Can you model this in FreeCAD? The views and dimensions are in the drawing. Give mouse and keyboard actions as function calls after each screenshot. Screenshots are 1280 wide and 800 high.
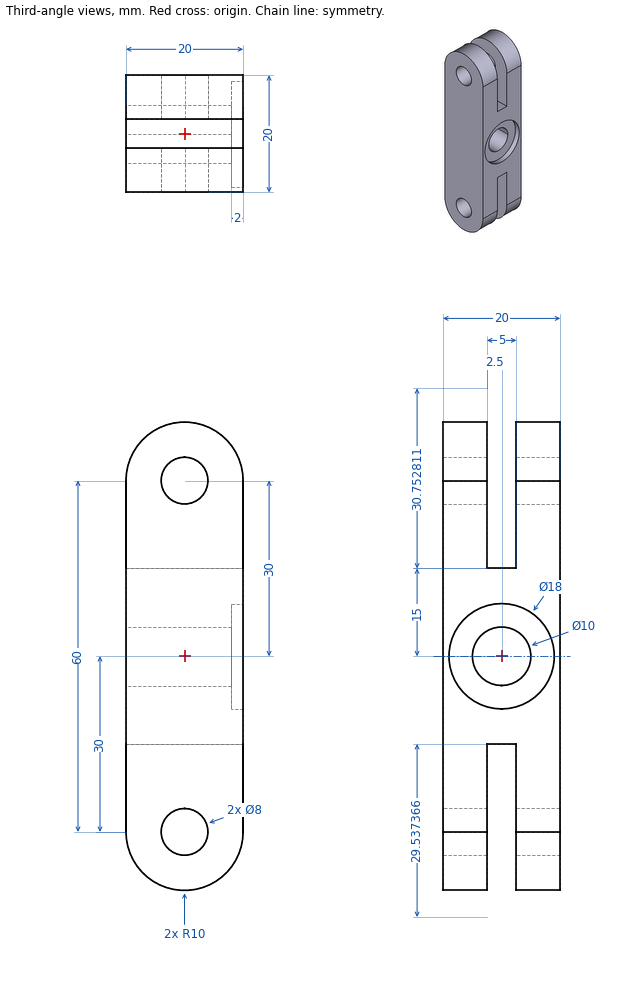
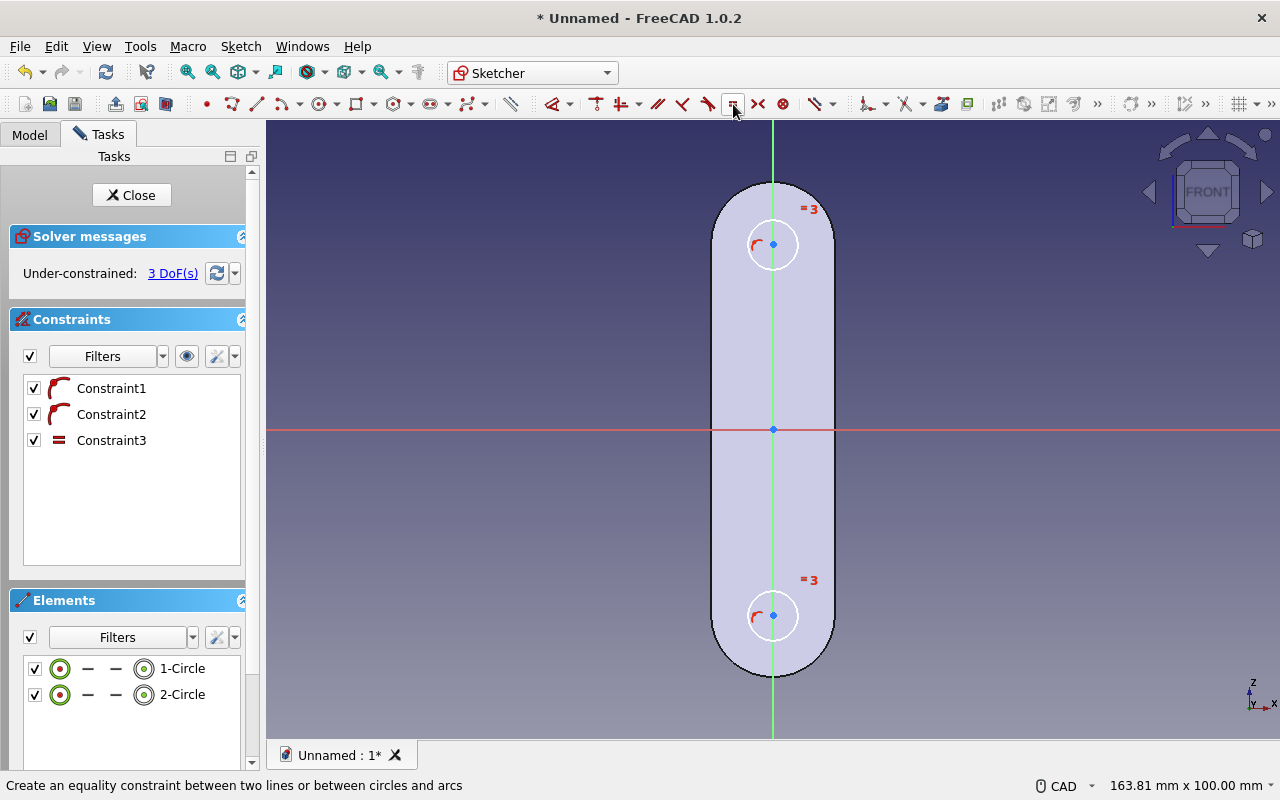
key(d)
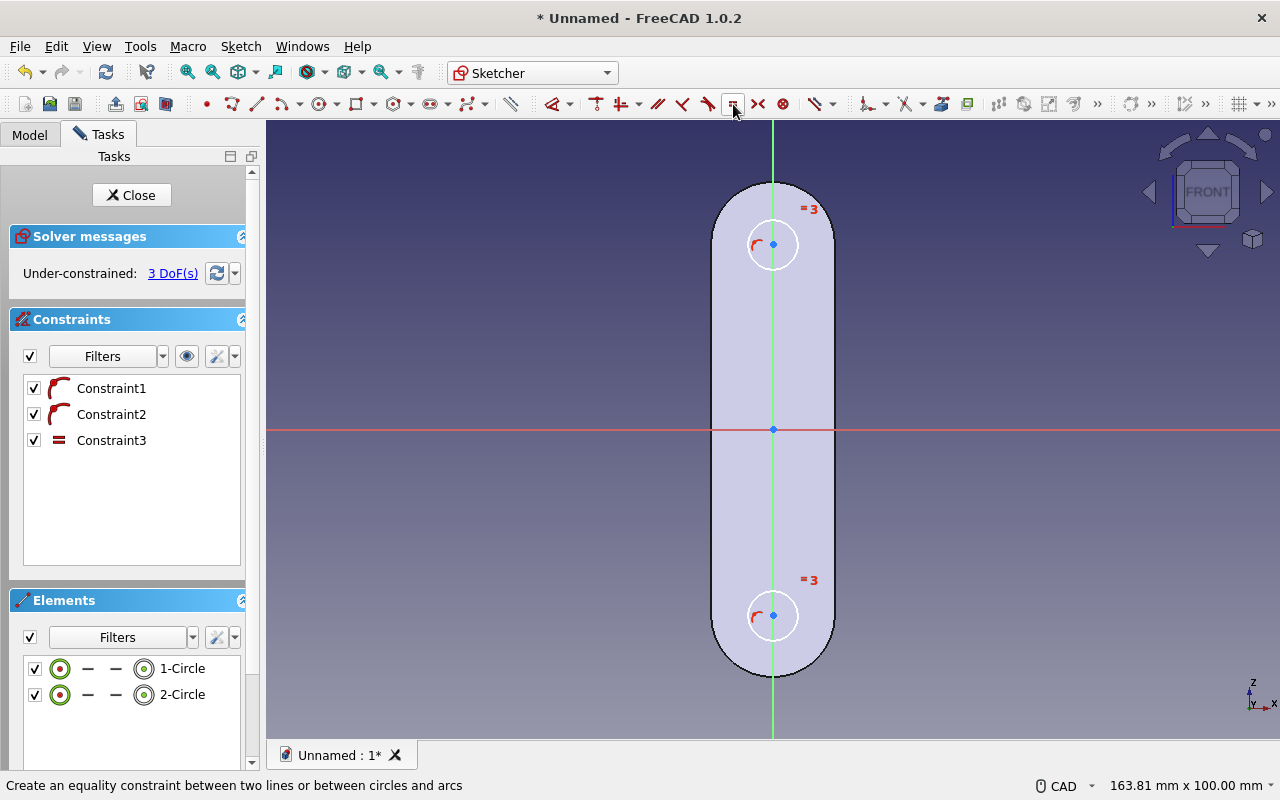
click(790, 598)
click(812, 575)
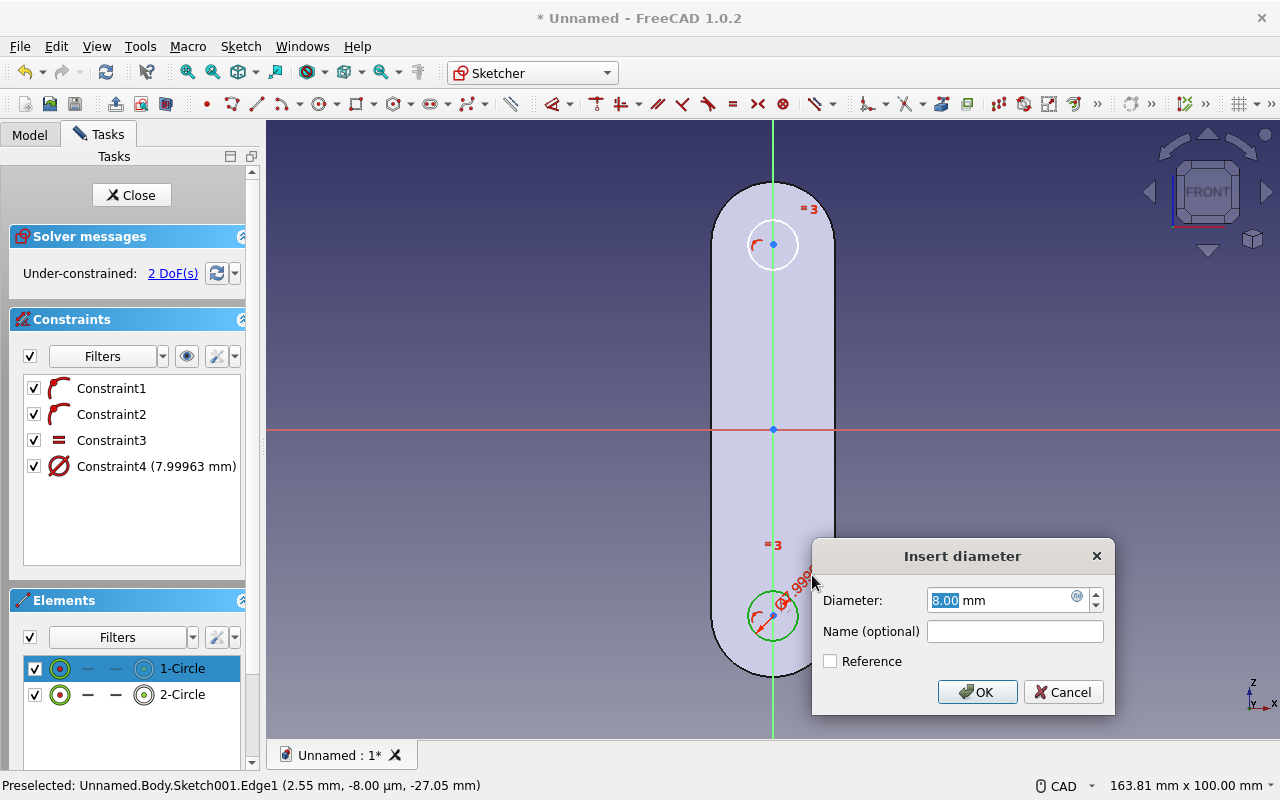
text(8)
key(Return)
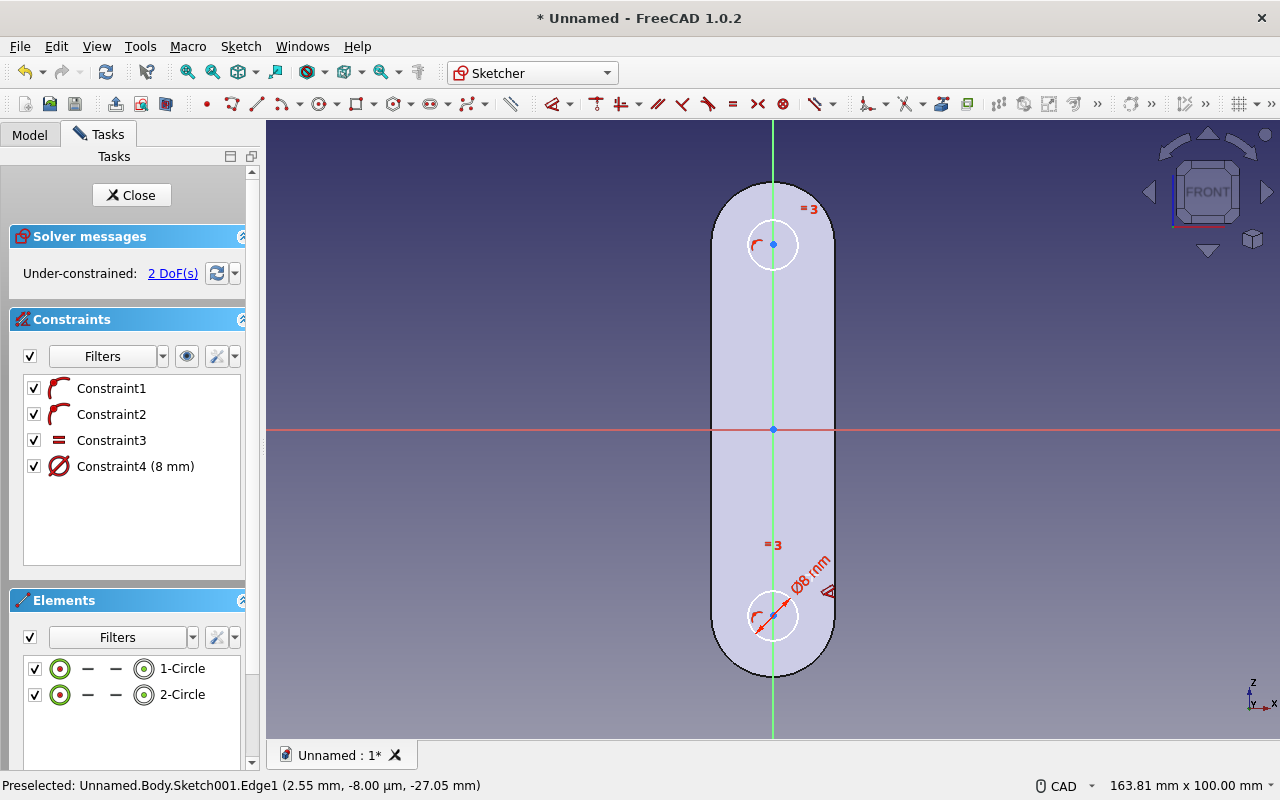
click(773, 616)
click(807, 523)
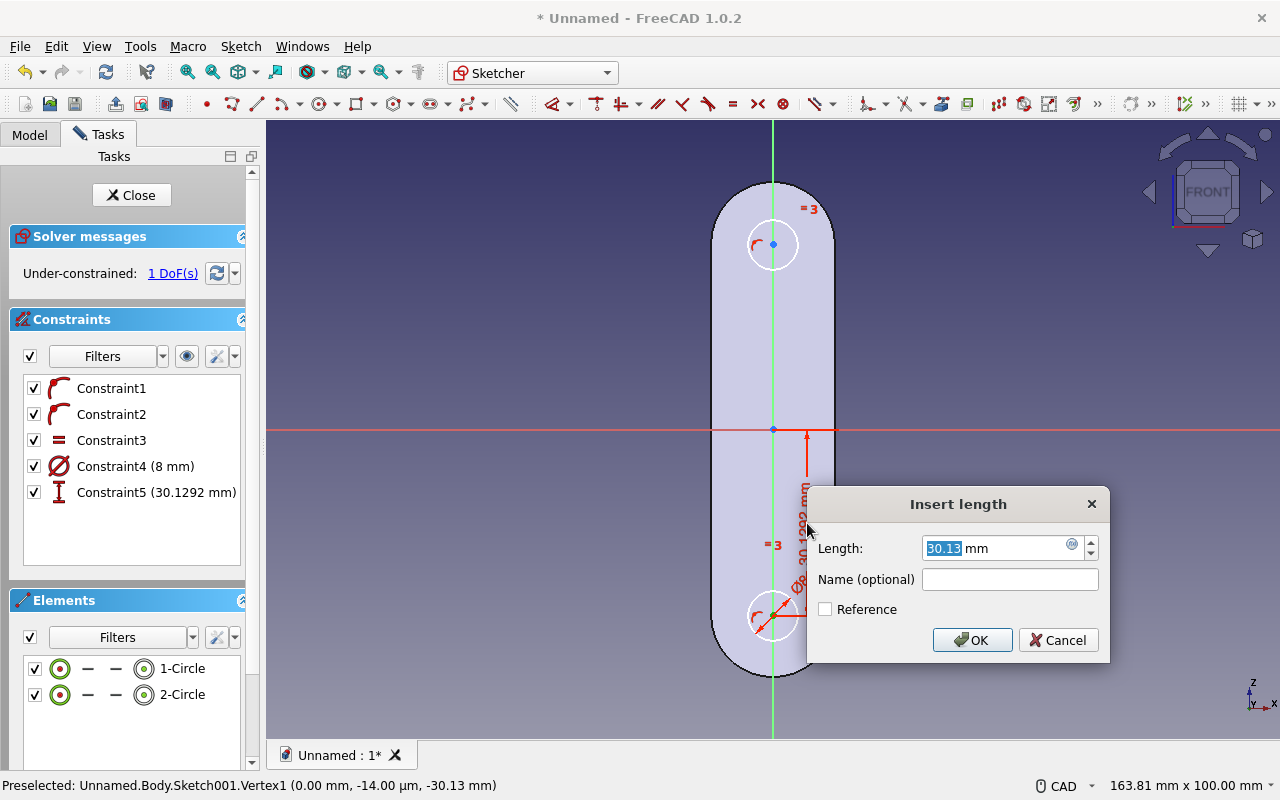
text(30)
key(Return)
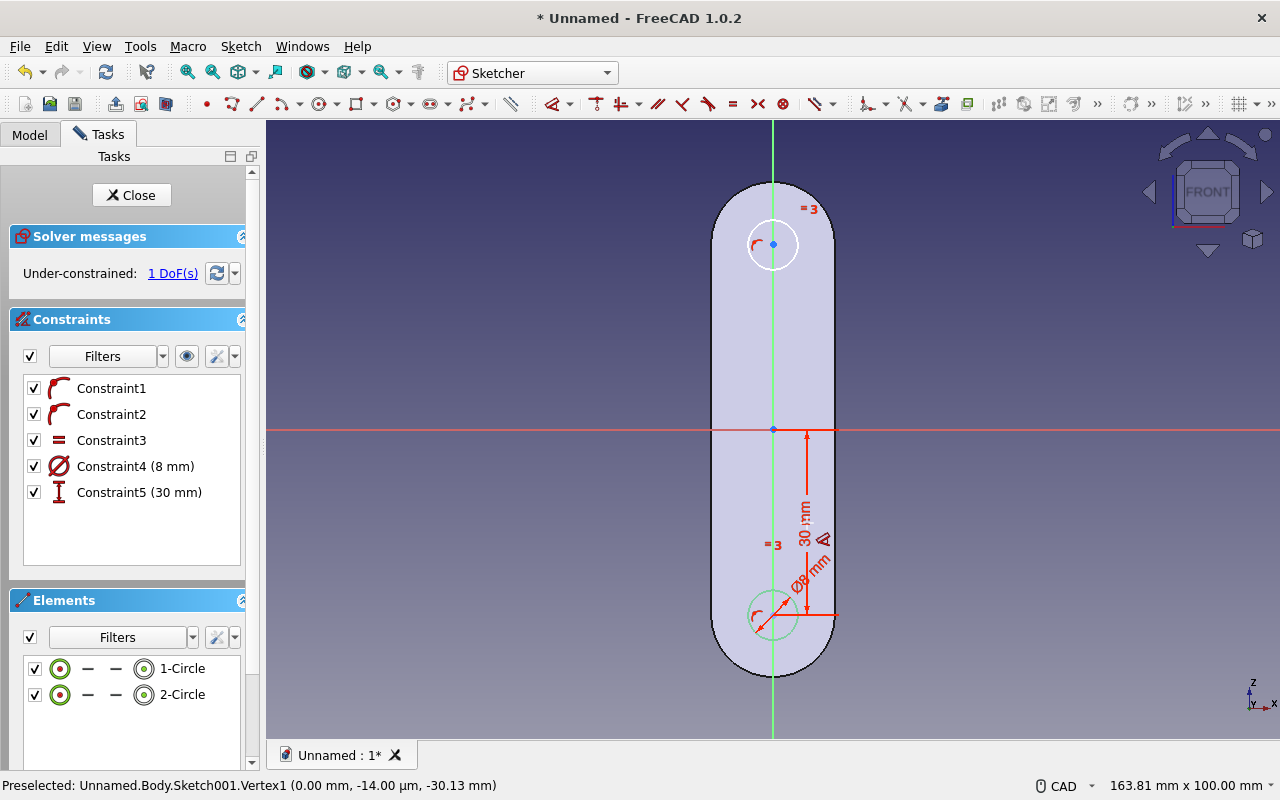
click(773, 245)
click(807, 337)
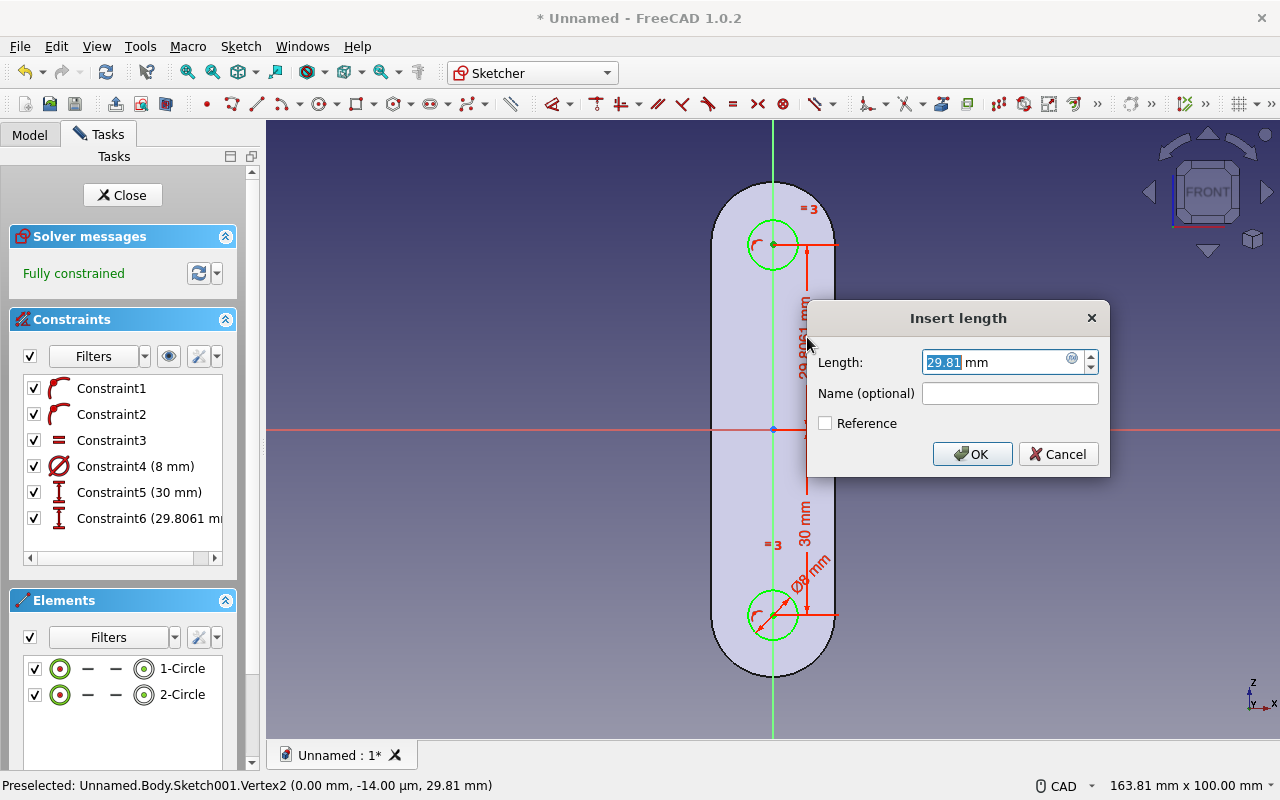
text(30)
key(Return)
key(Escape)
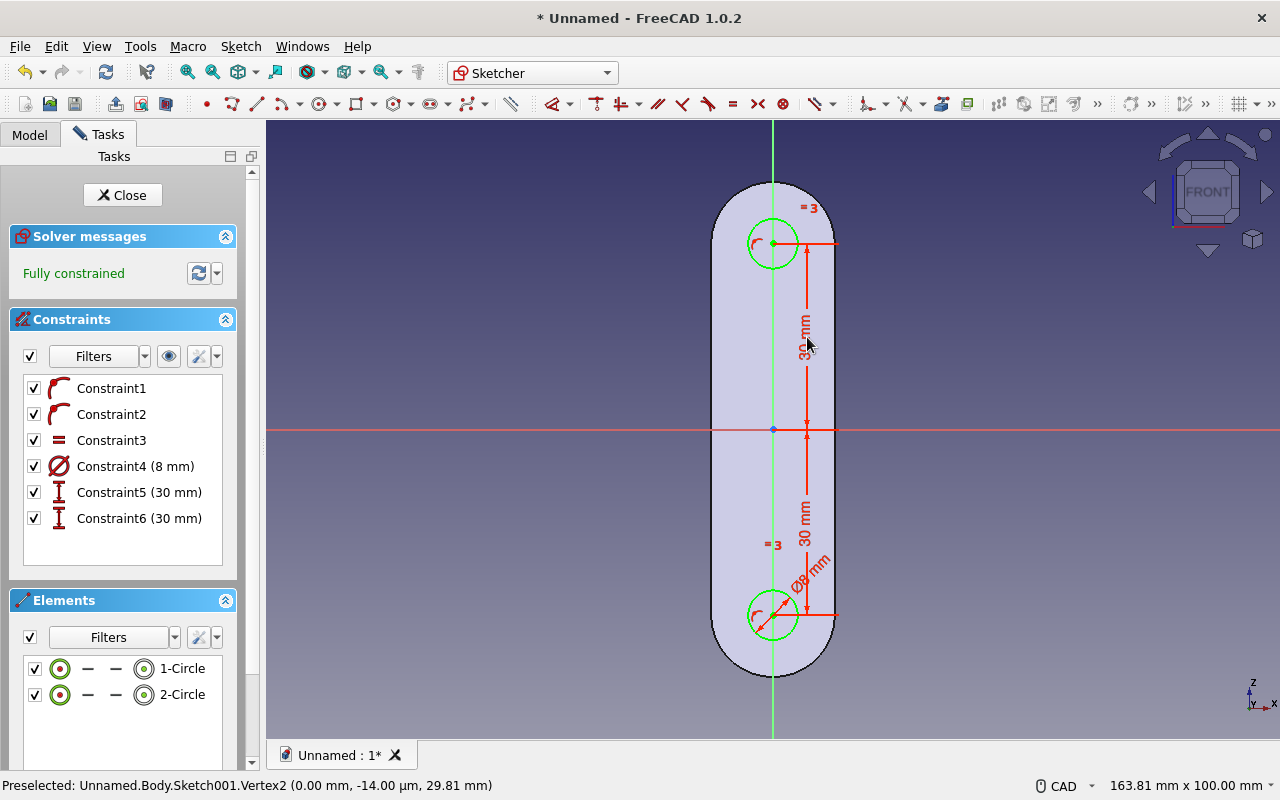
click(123, 195)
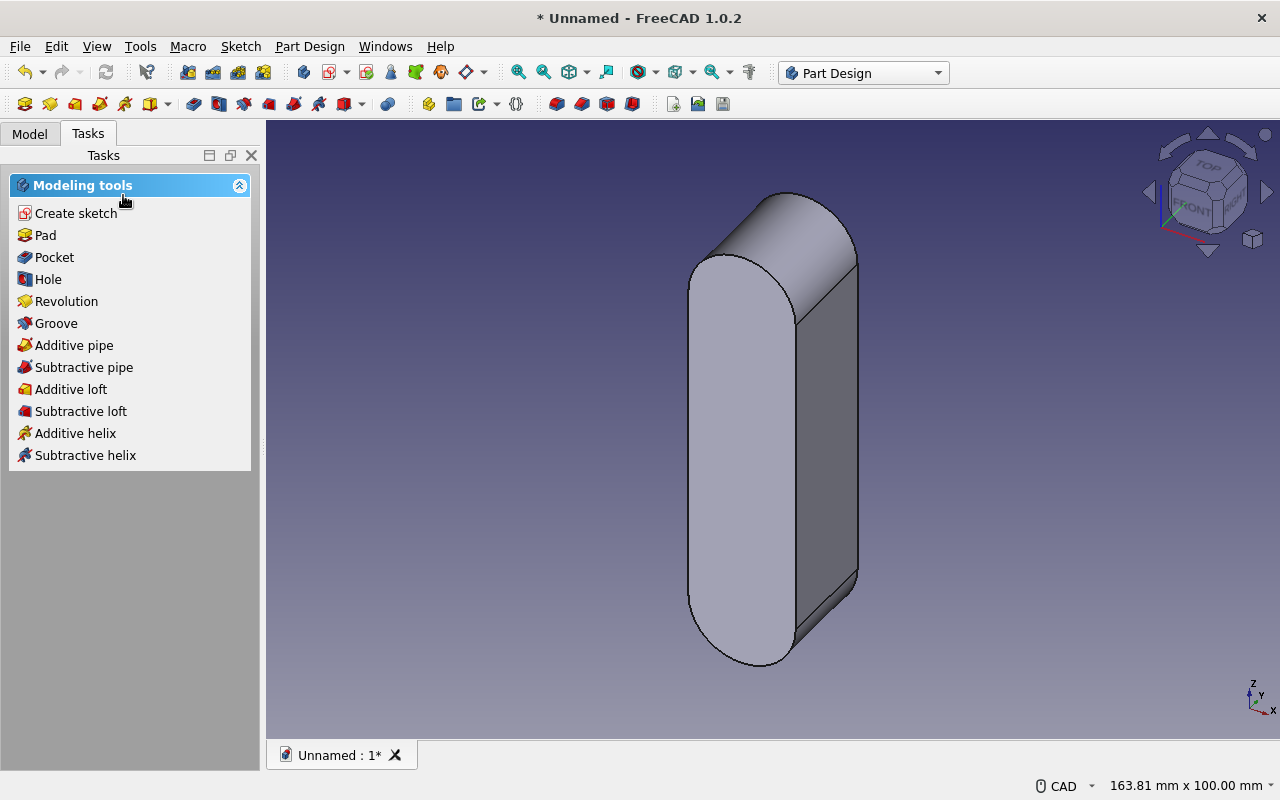
click(194, 104)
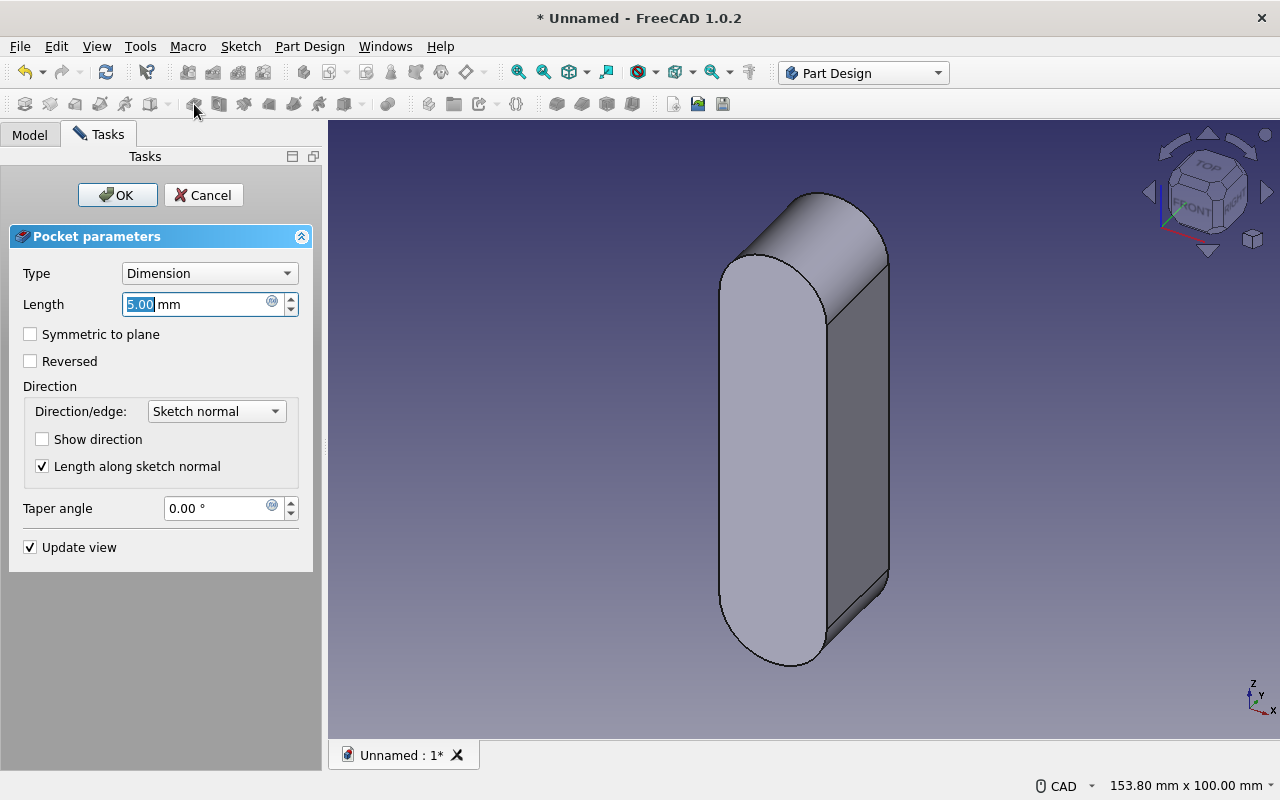
text(20)
key(Tab)